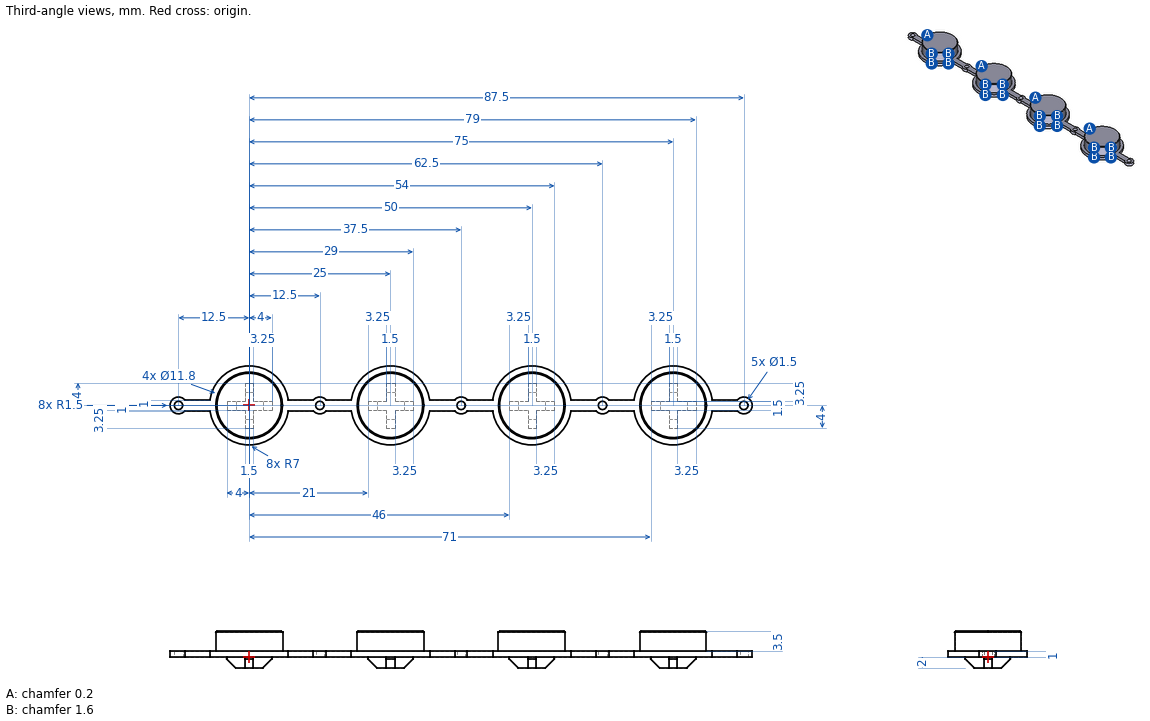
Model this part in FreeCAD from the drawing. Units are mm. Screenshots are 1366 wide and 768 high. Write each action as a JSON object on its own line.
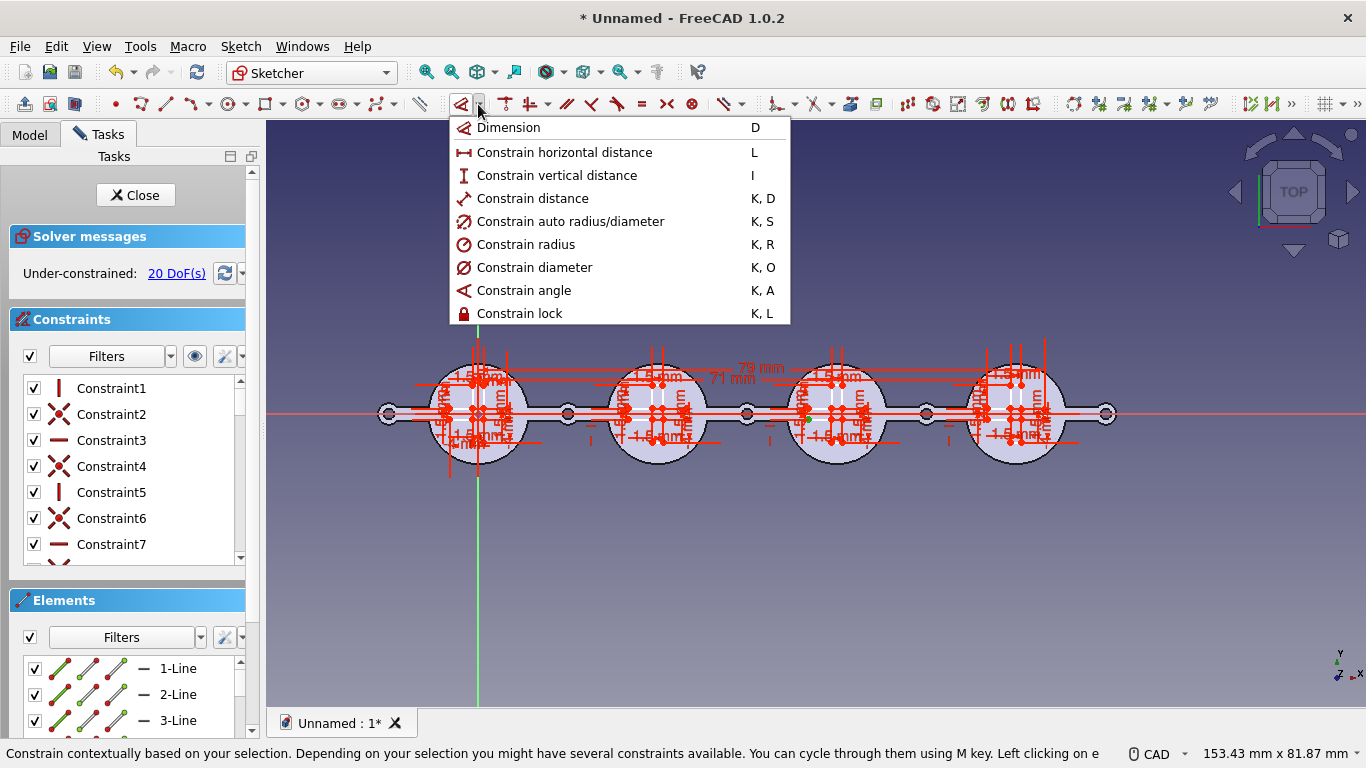
{"action": "left_click", "coordinate": [620, 152]}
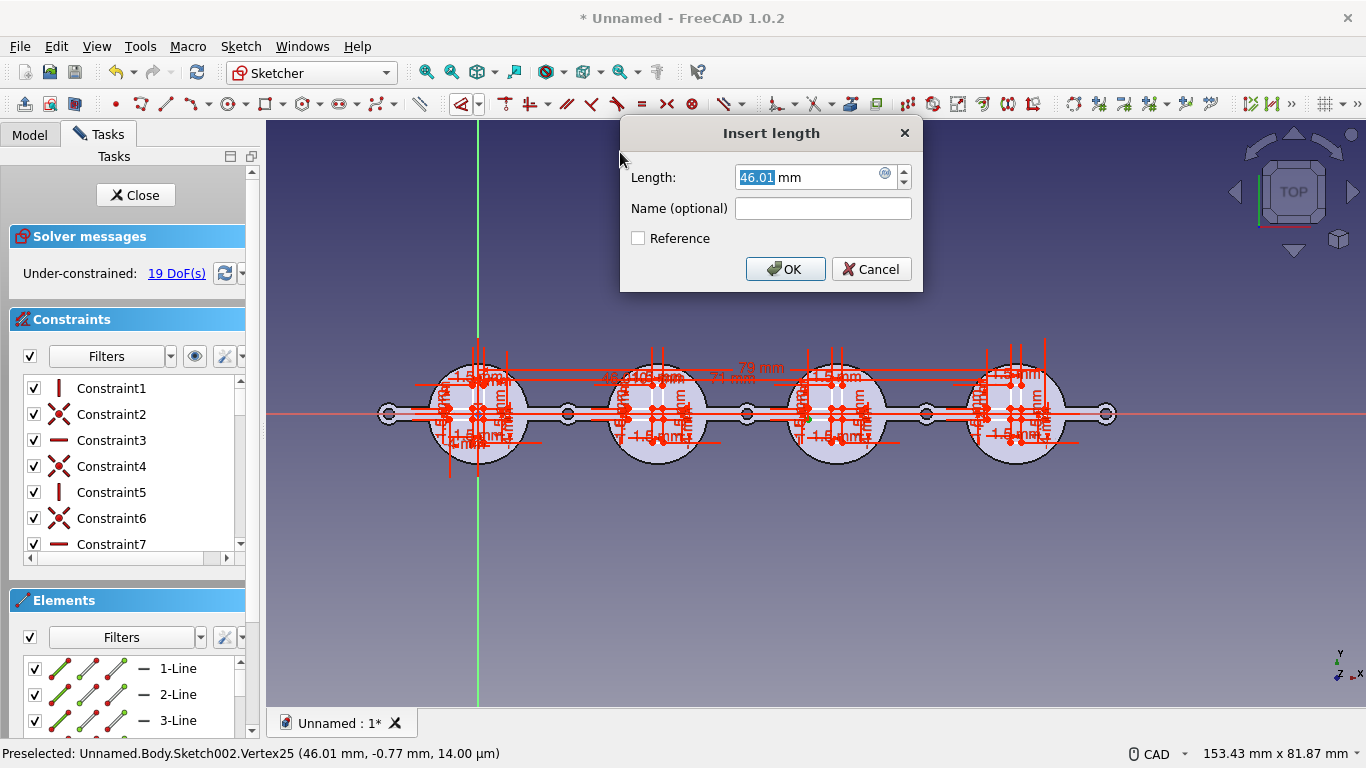
{"action": "type", "text": "46"}
{"action": "key", "text": "Return"}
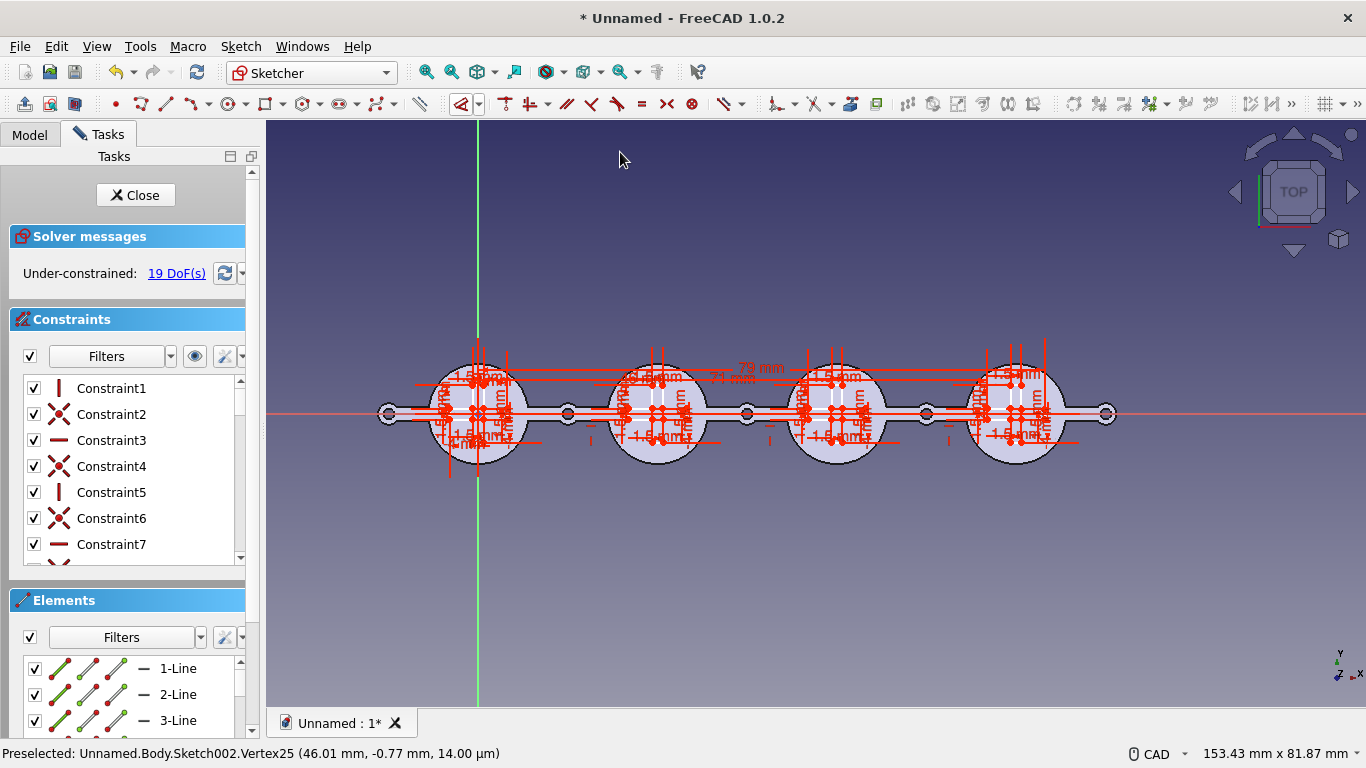
{"action": "left_click", "coordinate": [866, 409]}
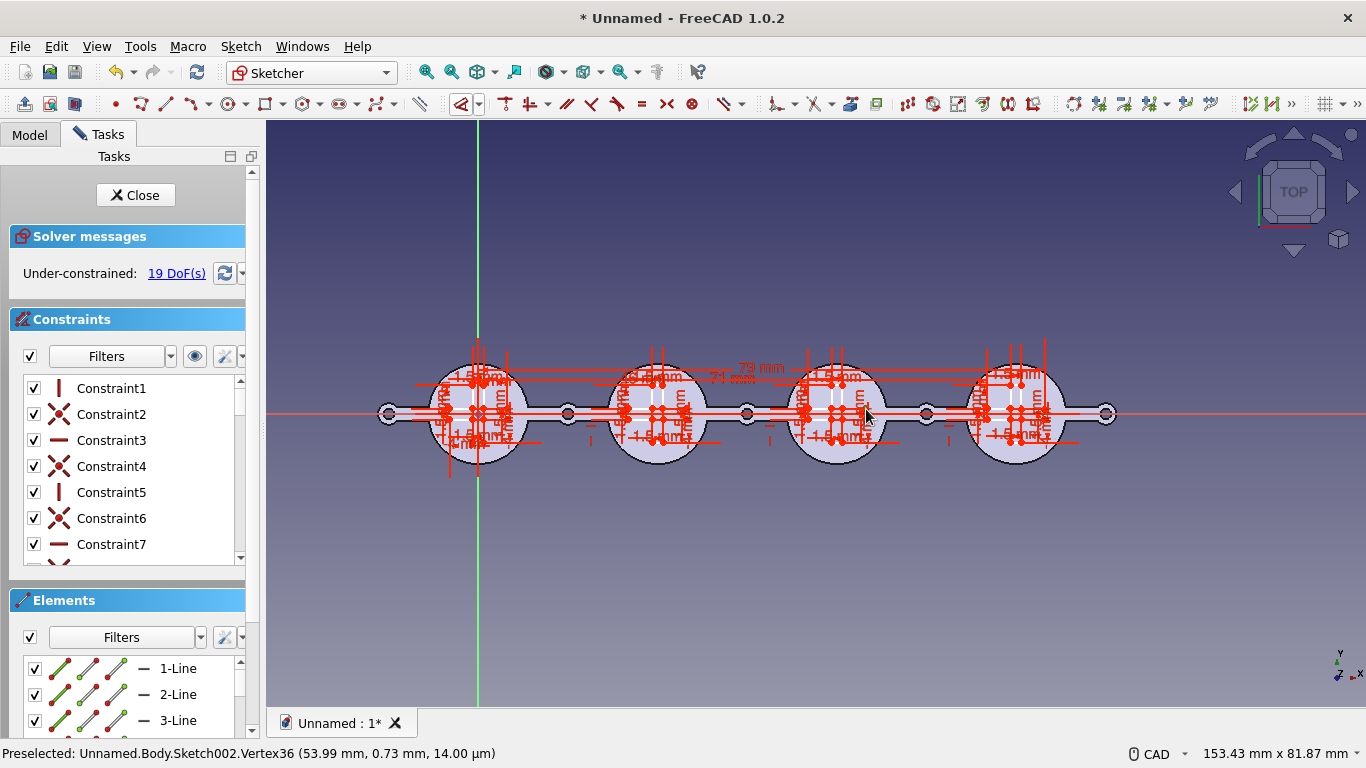
{"action": "key", "text": "l"}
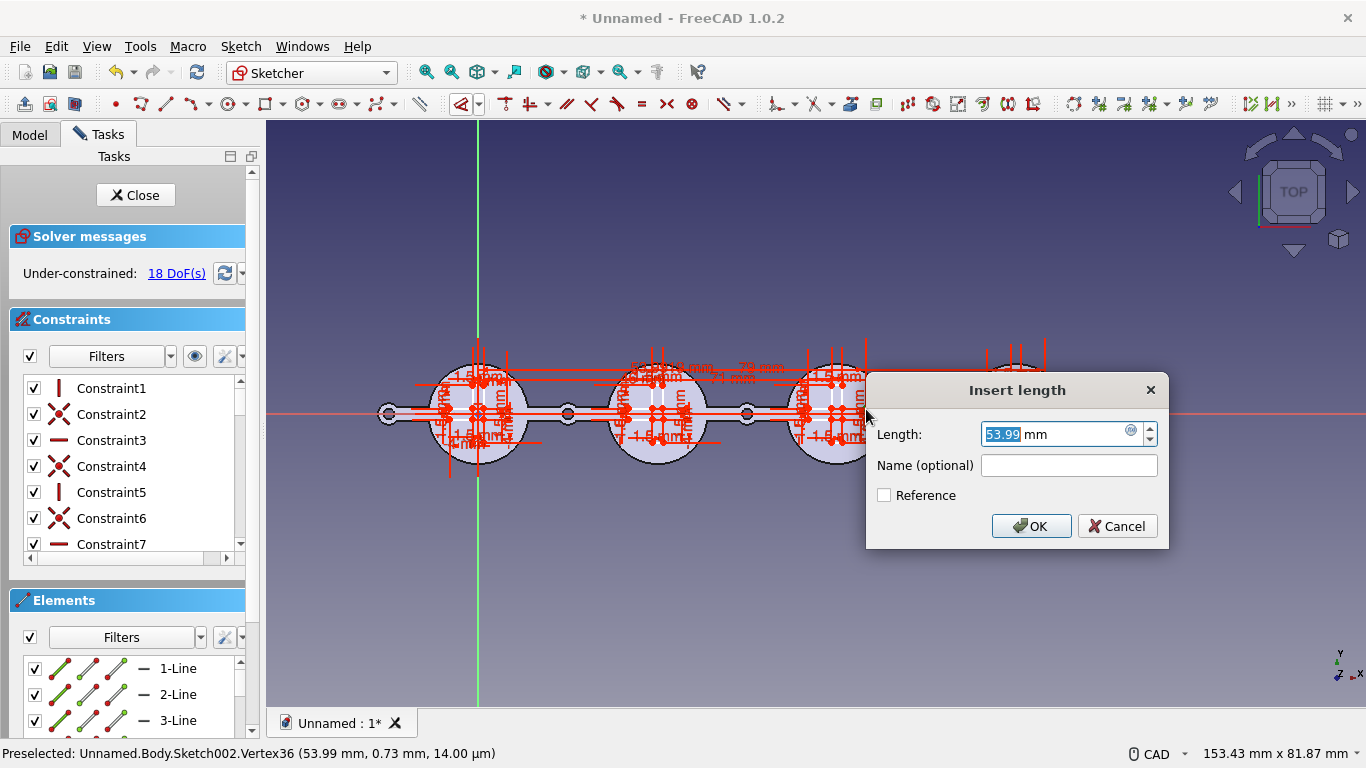
{"action": "type", "text": "54"}
{"action": "key", "text": "Return"}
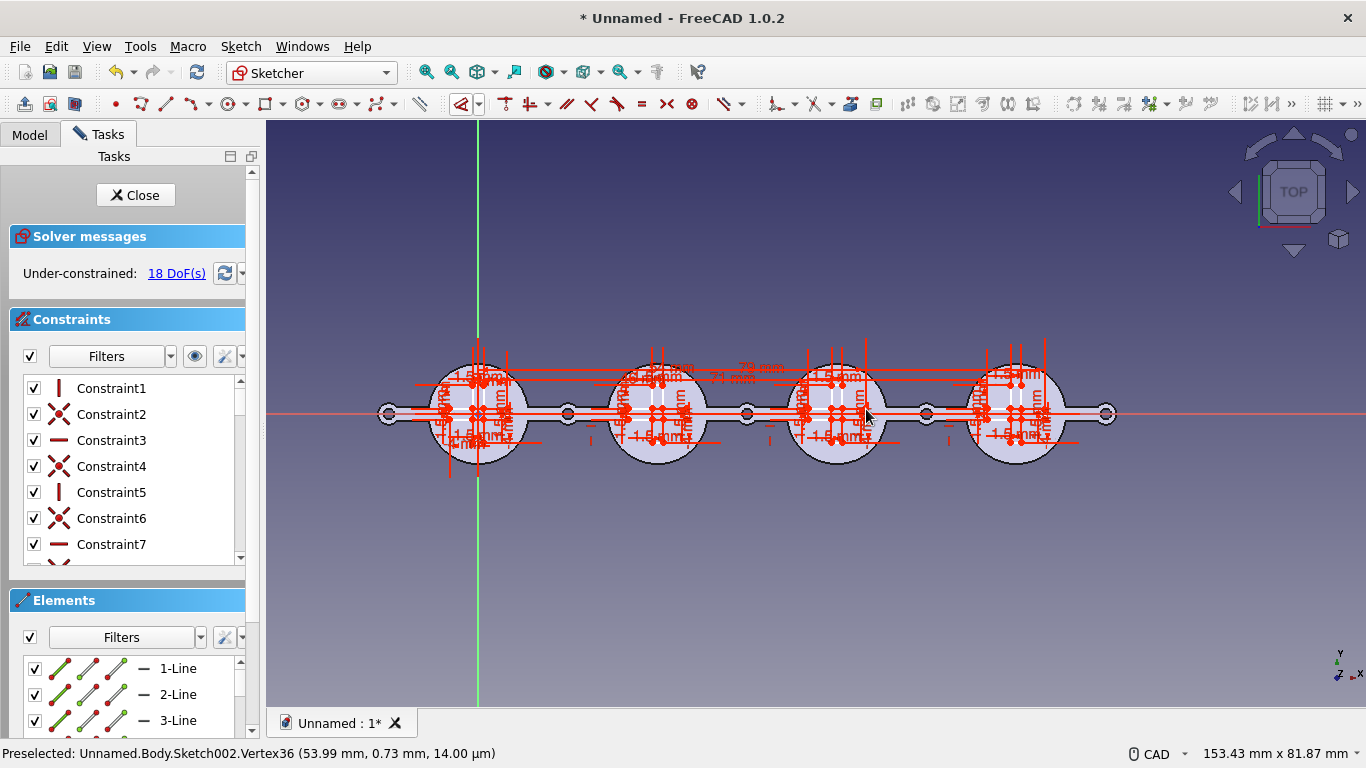
{"action": "left_click", "coordinate": [629, 420]}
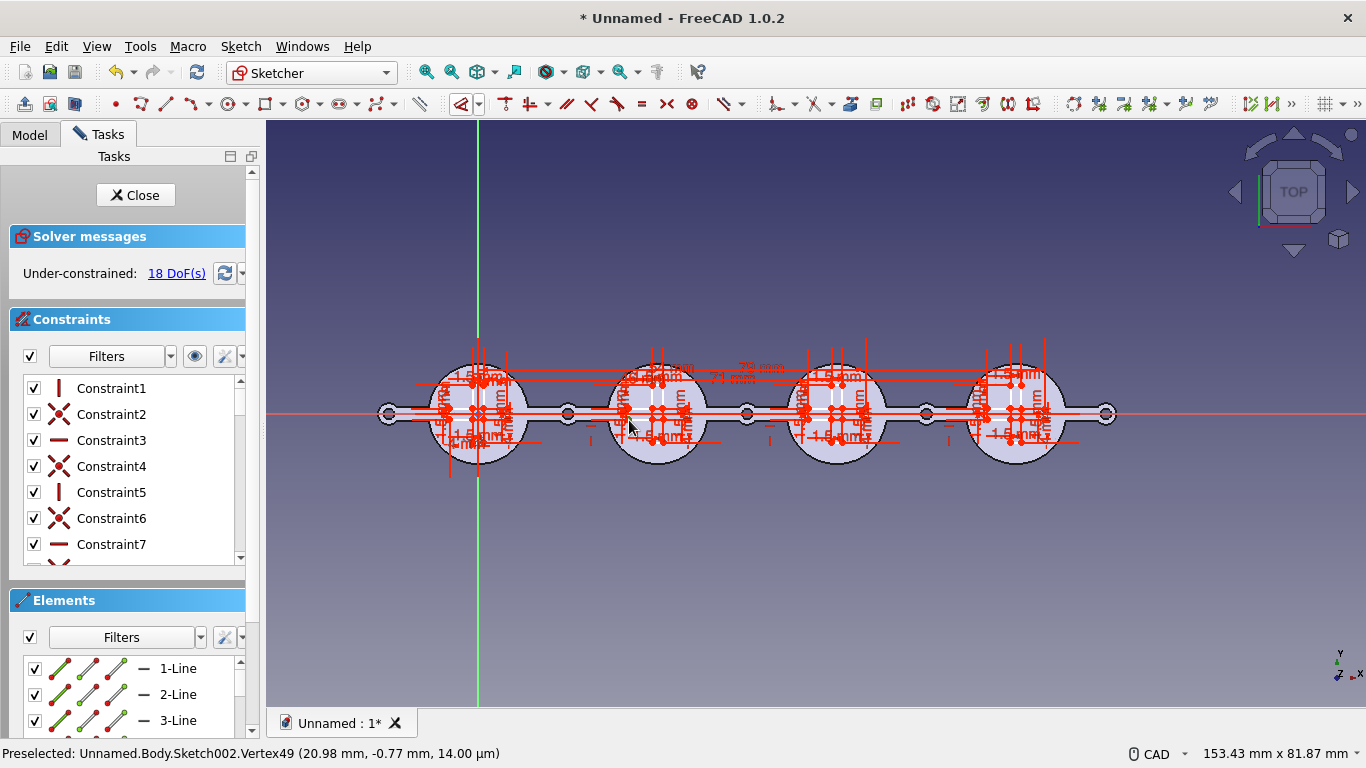
{"action": "key", "text": "l"}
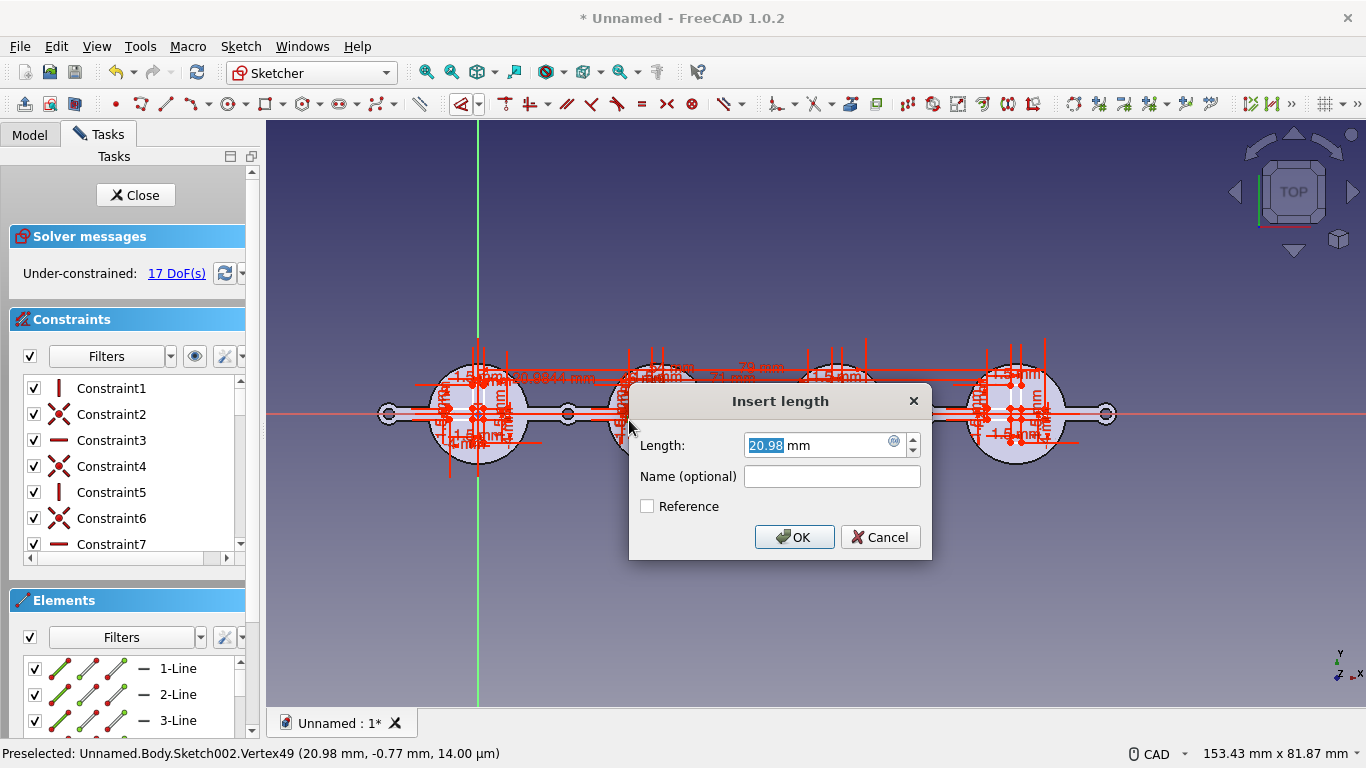
{"action": "type", "text": "21"}
{"action": "key", "text": "Return"}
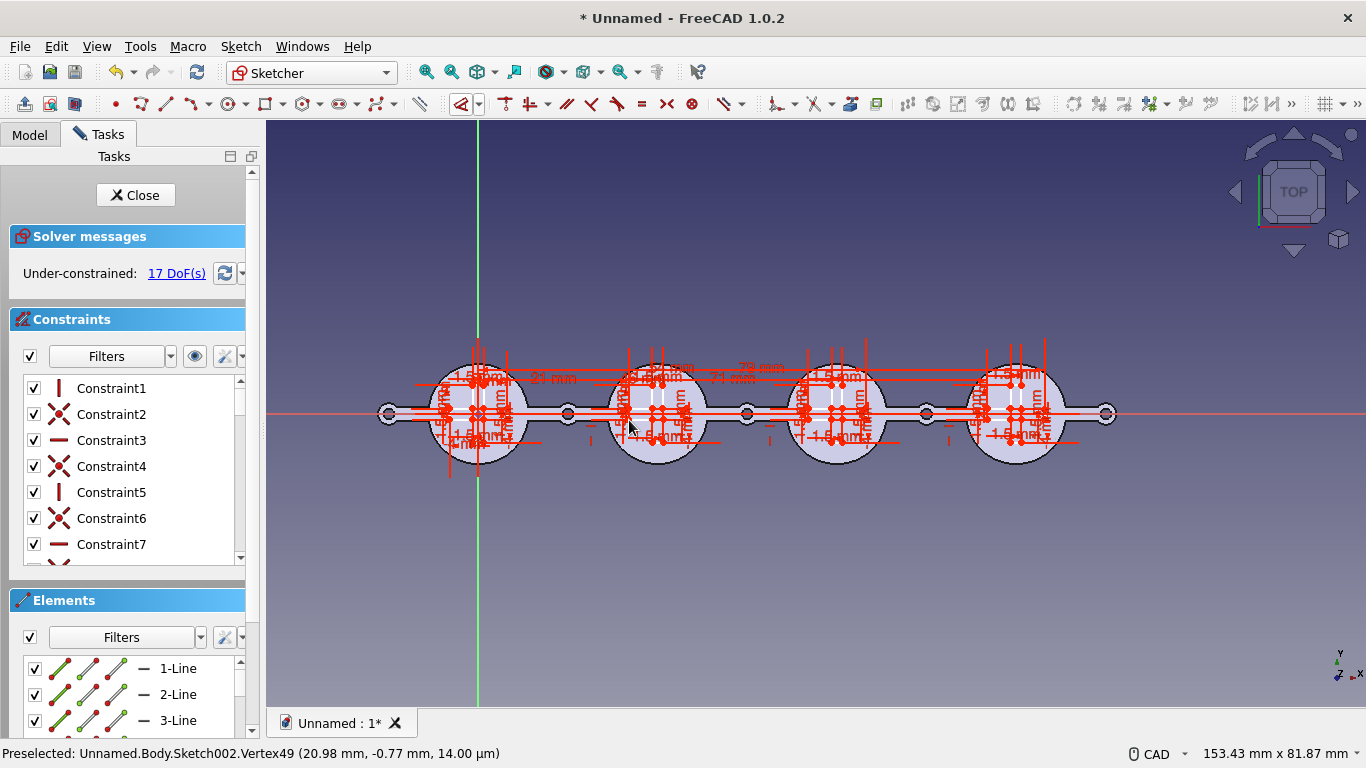
{"action": "left_click", "coordinate": [686, 409]}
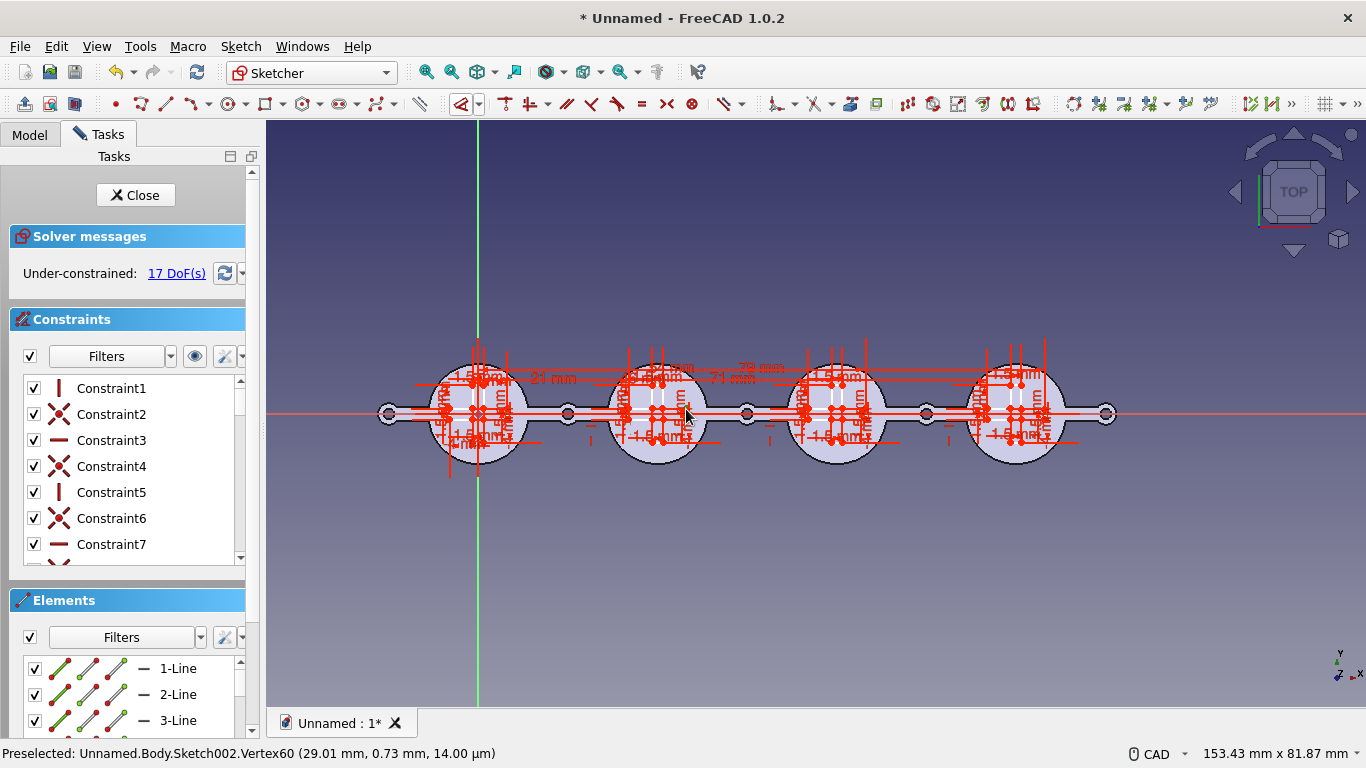
{"action": "key", "text": "l"}